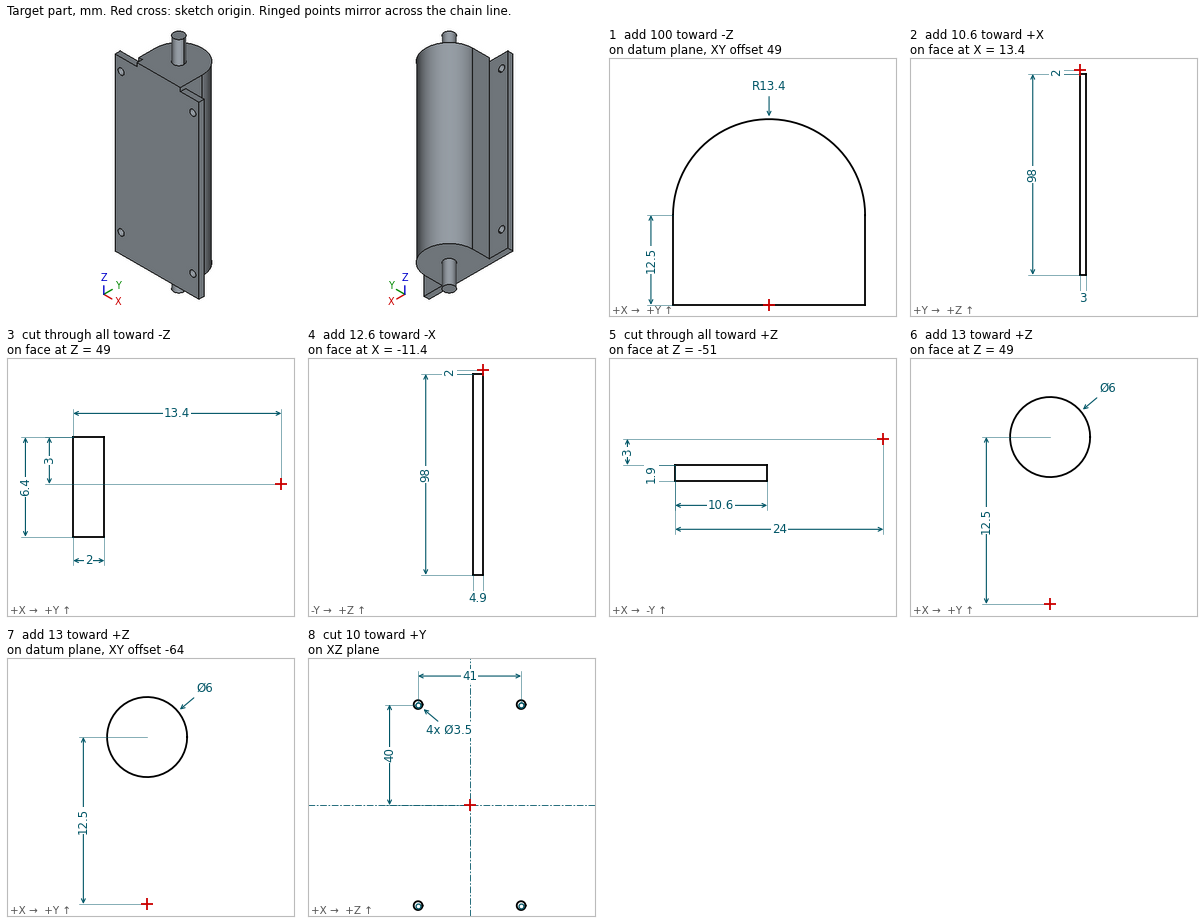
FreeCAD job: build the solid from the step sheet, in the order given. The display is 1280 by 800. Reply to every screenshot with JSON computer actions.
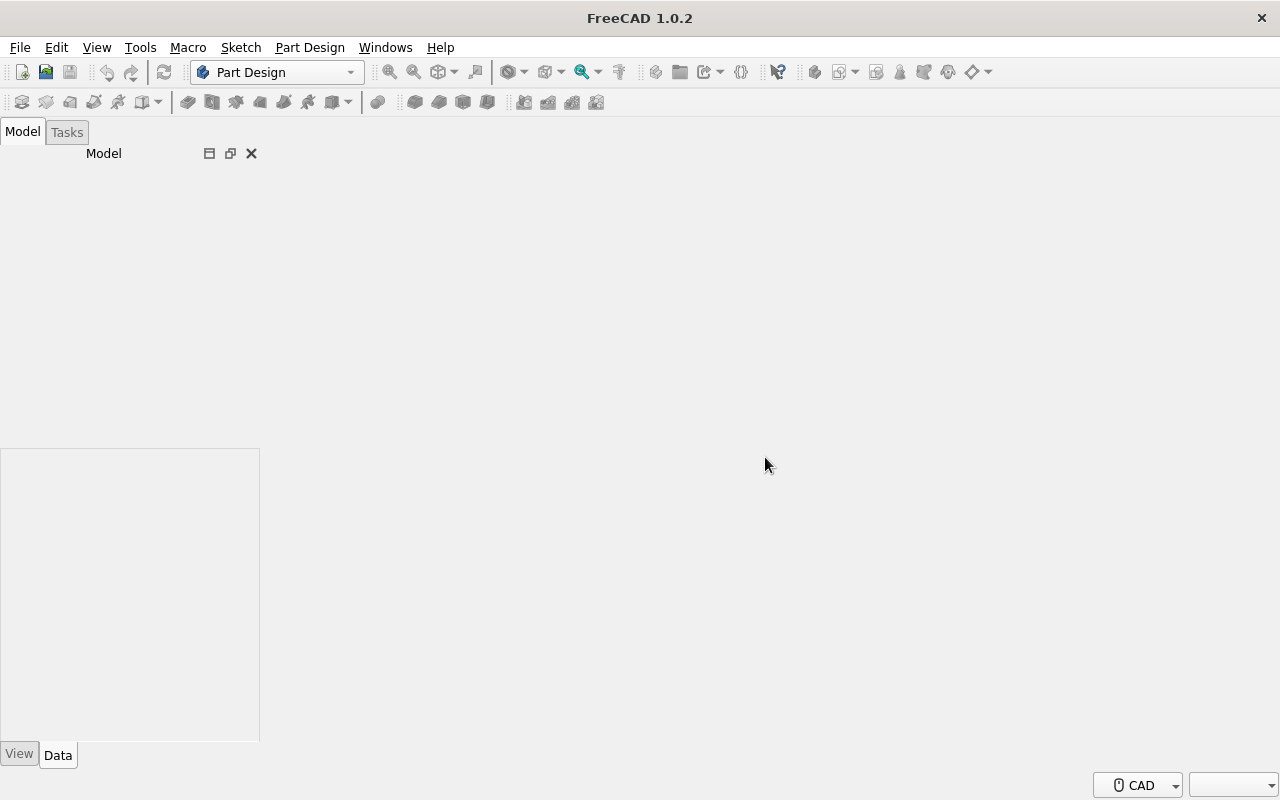
{"action": "left_click", "coordinate": [22, 72]}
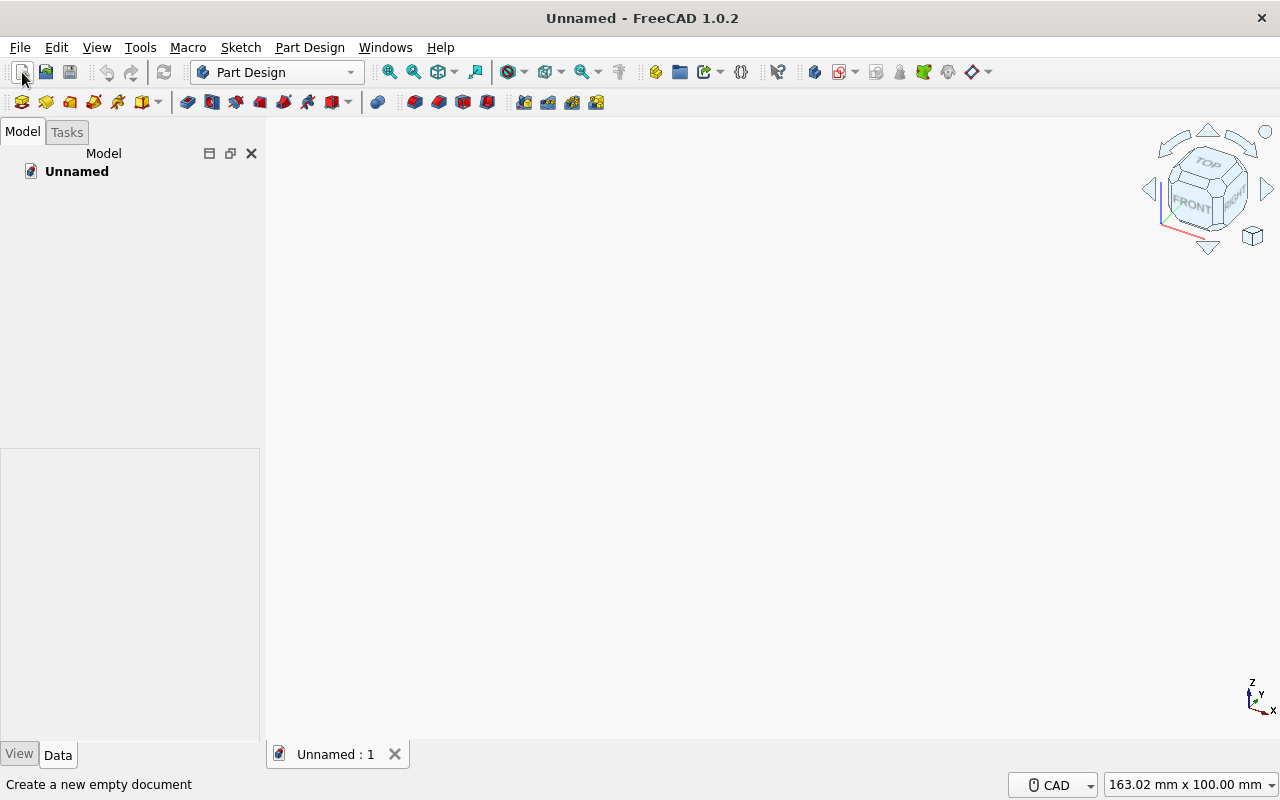
{"action": "left_click", "coordinate": [816, 72]}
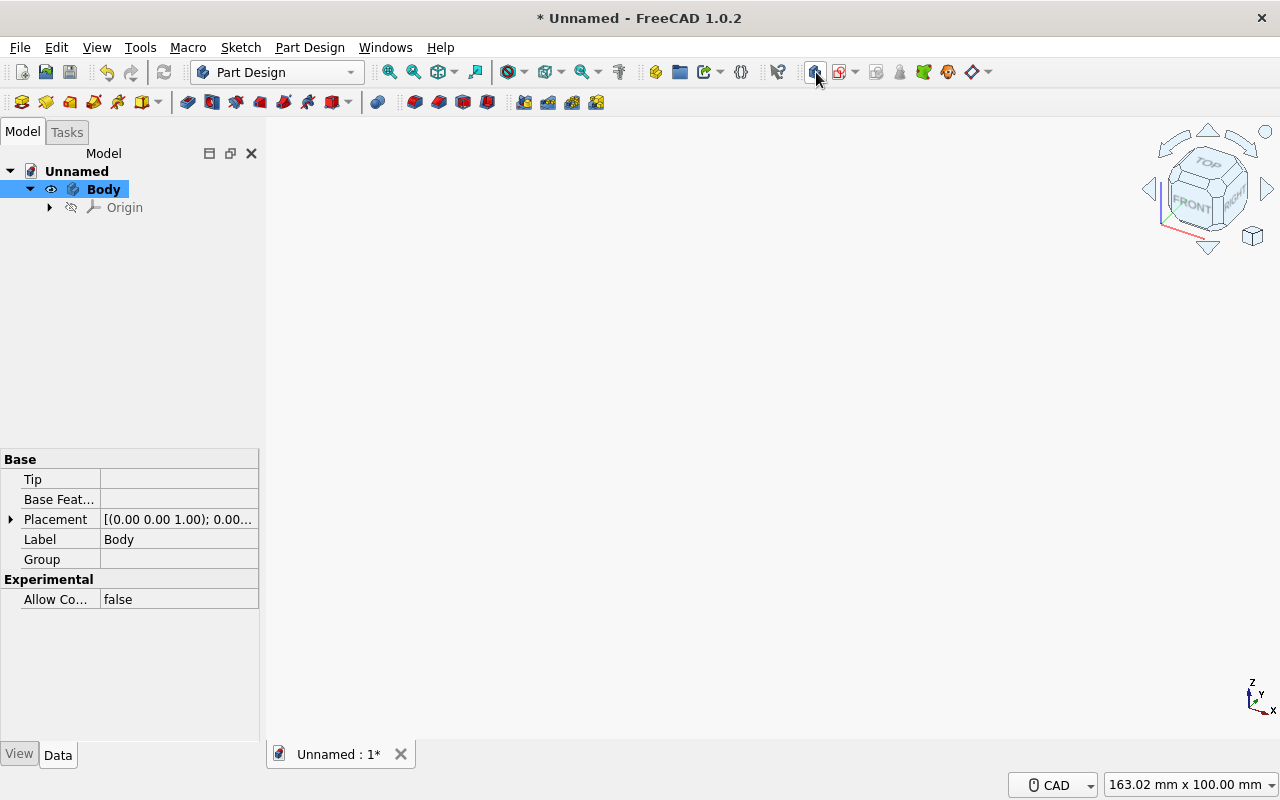
{"action": "left_click", "coordinate": [50, 207]}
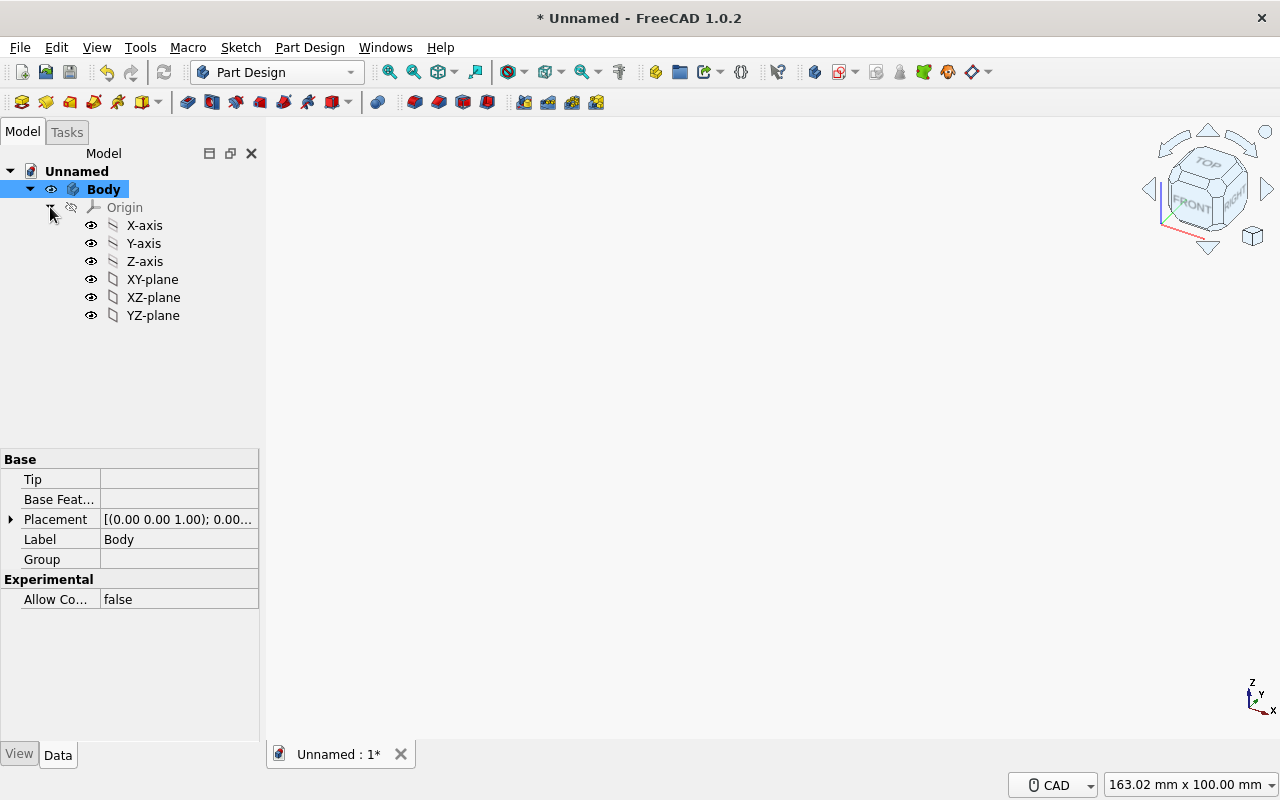
{"action": "left_click", "coordinate": [136, 279]}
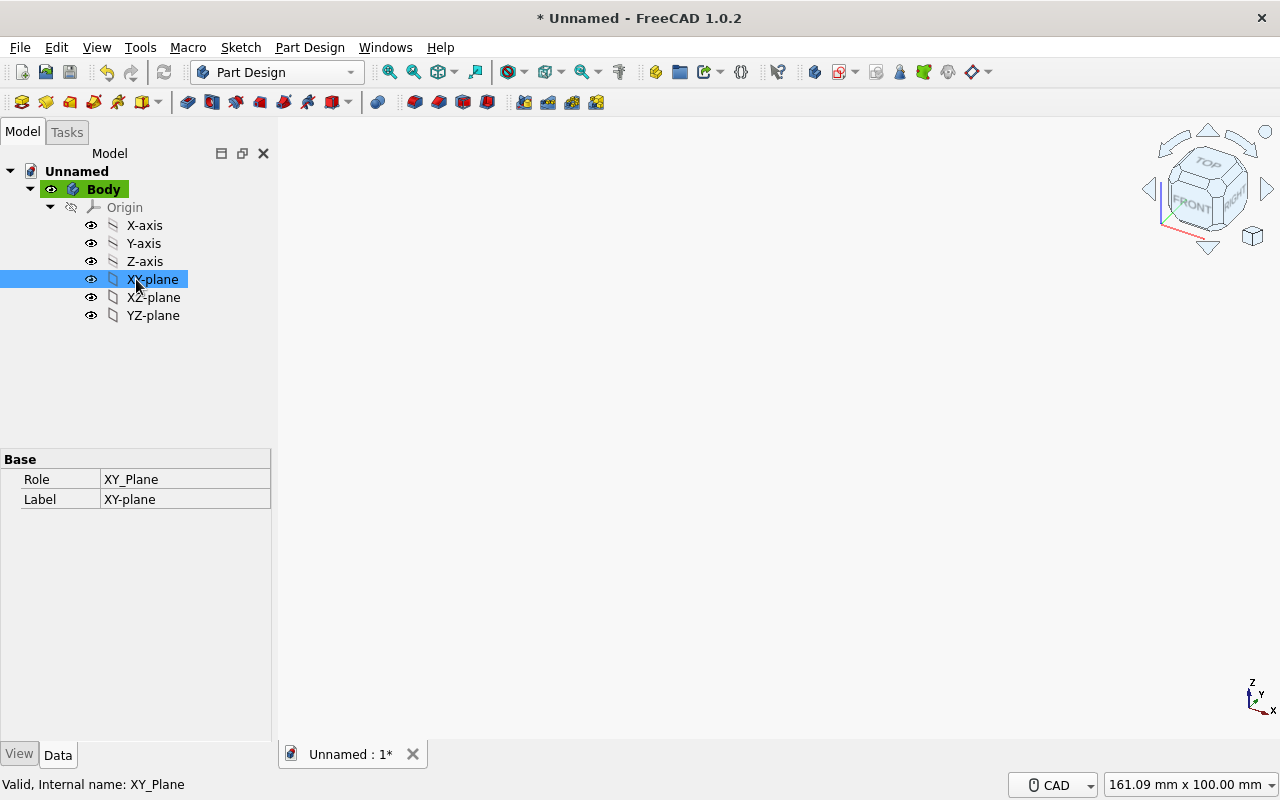
{"action": "left_click", "coordinate": [972, 72]}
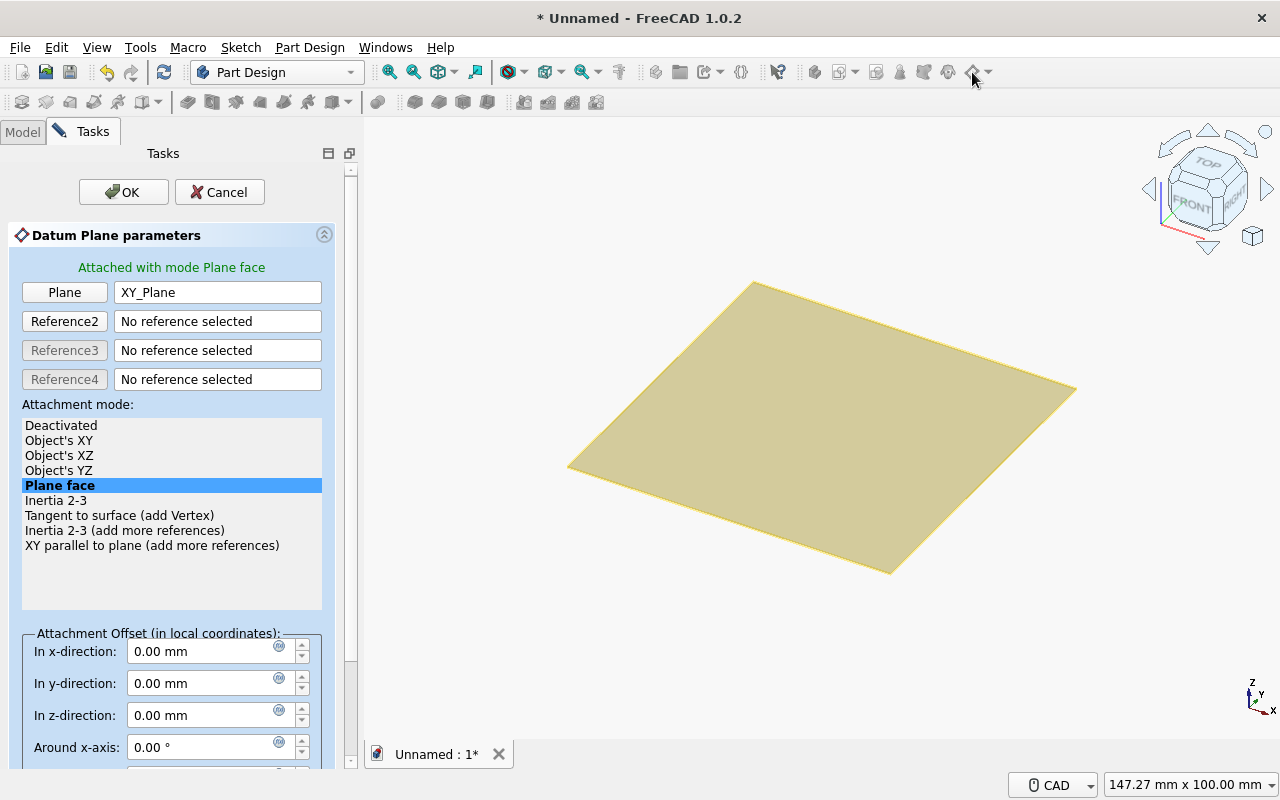
{"action": "triple_click", "coordinate": [210, 715]}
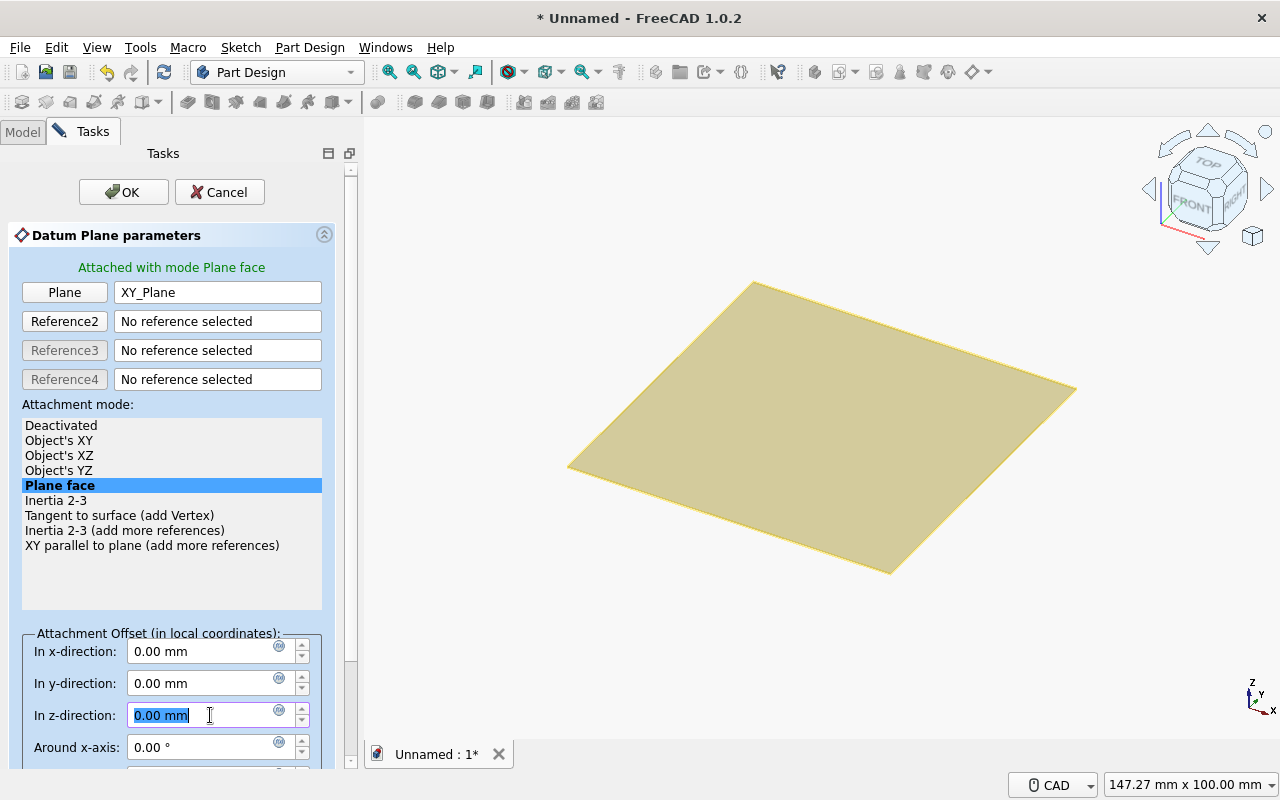
{"action": "type", "text": "49"}
{"action": "key", "text": "Tab"}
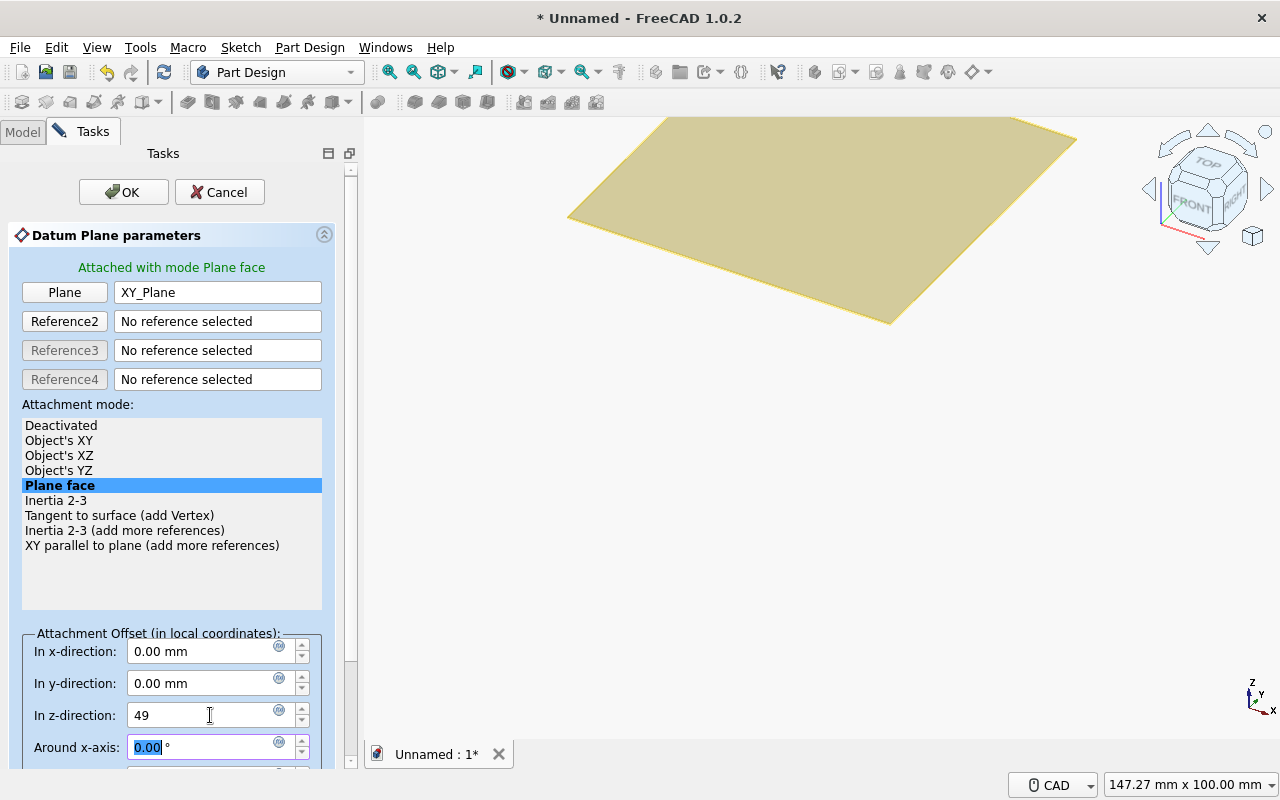
{"action": "left_click", "coordinate": [124, 192]}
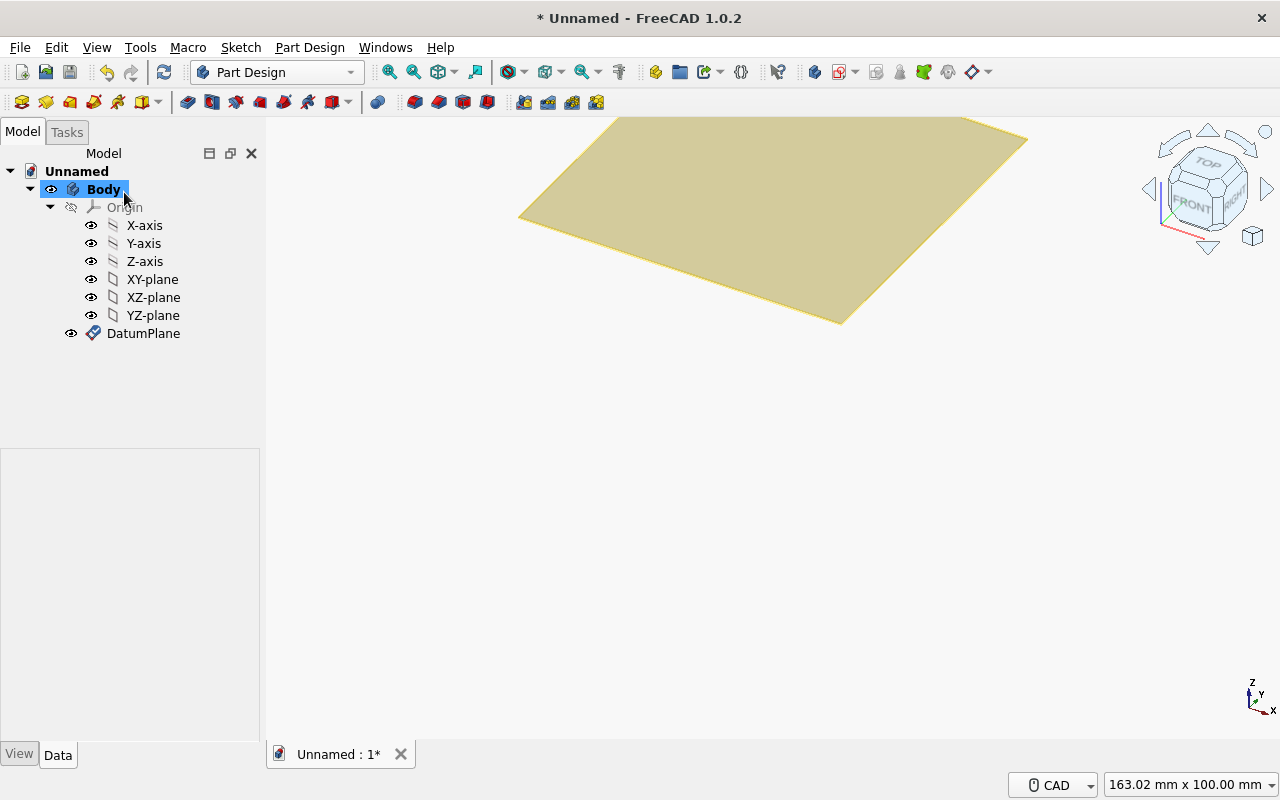
{"action": "left_click", "coordinate": [116, 333]}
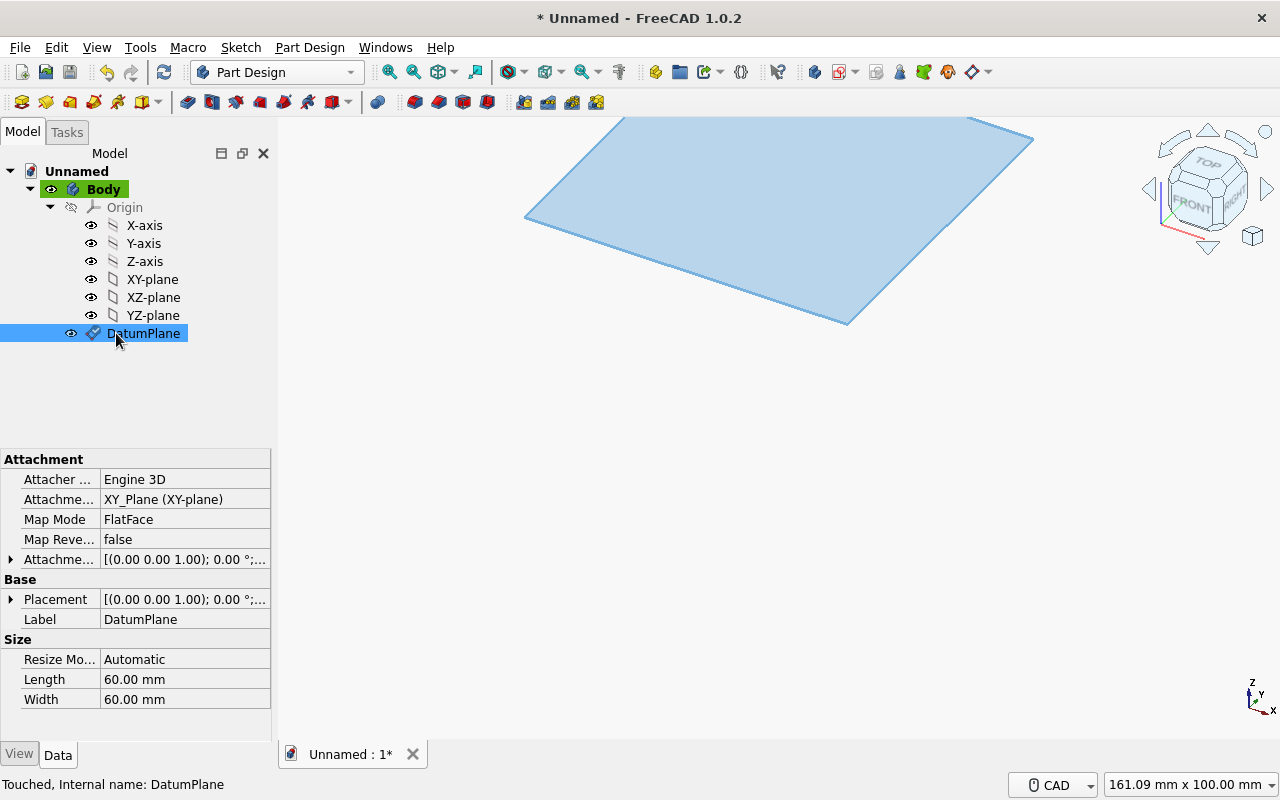
{"action": "left_click", "coordinate": [840, 72]}